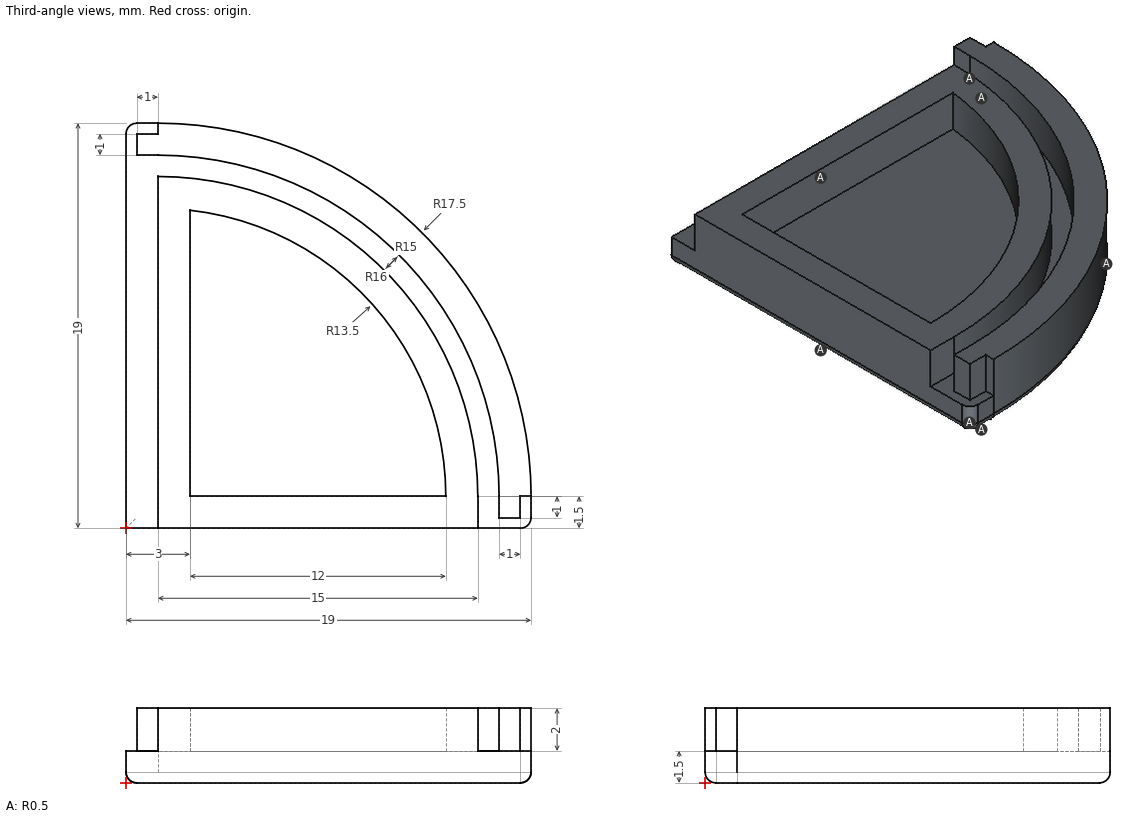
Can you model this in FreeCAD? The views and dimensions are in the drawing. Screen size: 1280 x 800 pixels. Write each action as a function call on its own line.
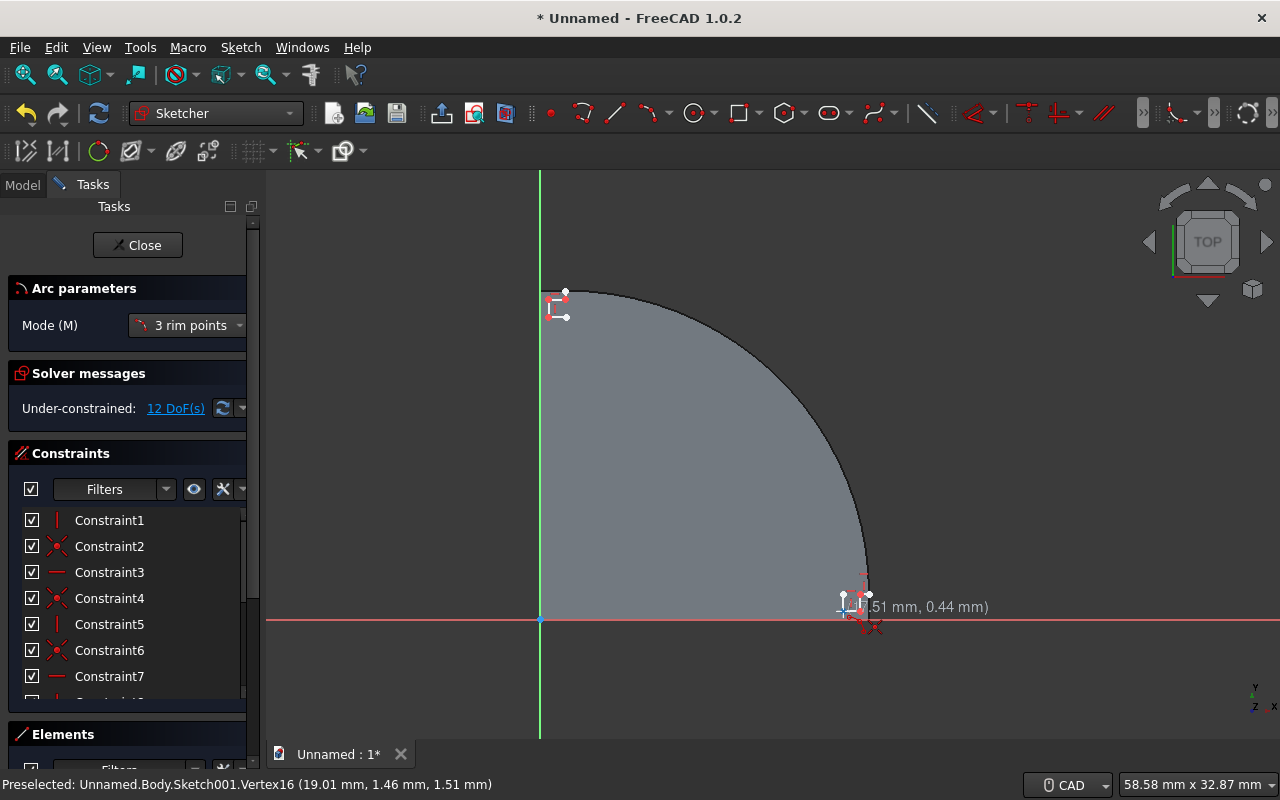
scroll(566, 317, up, 4)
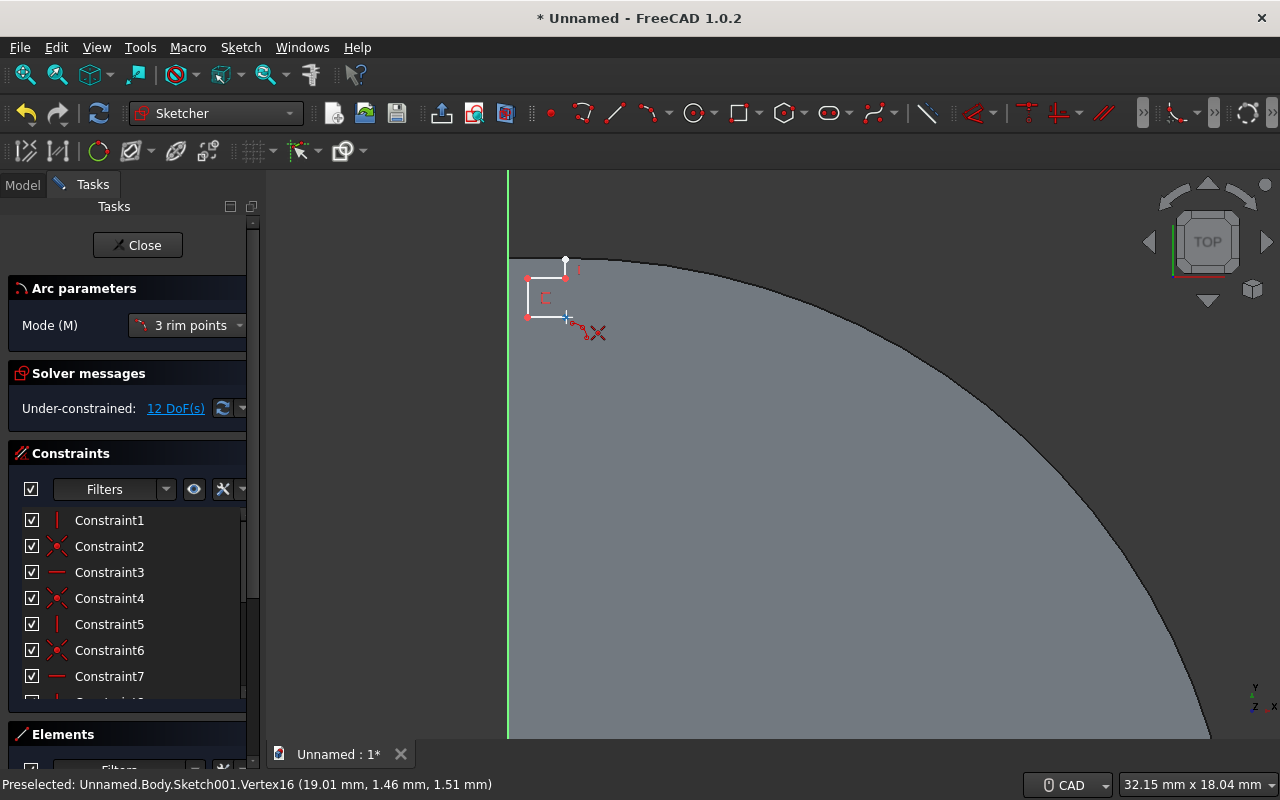
click(566, 317)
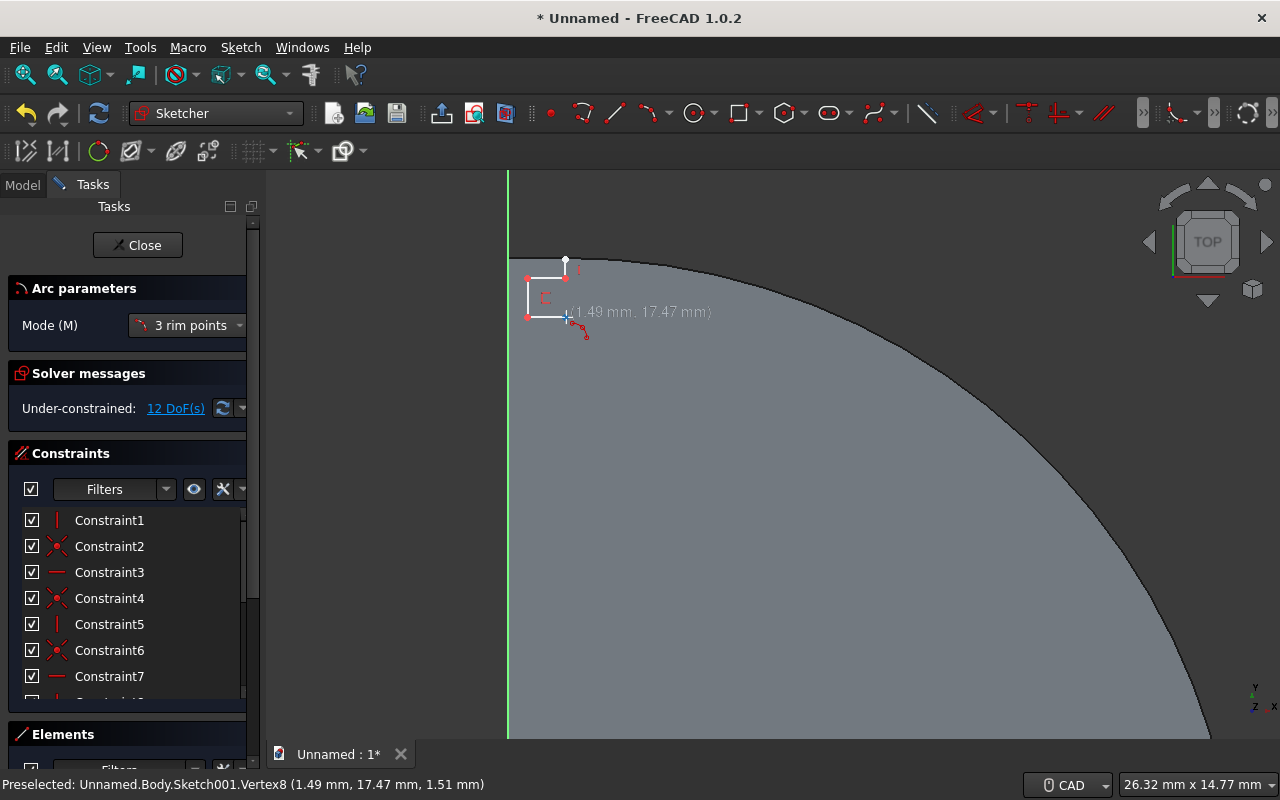
scroll(566, 316, down, 4)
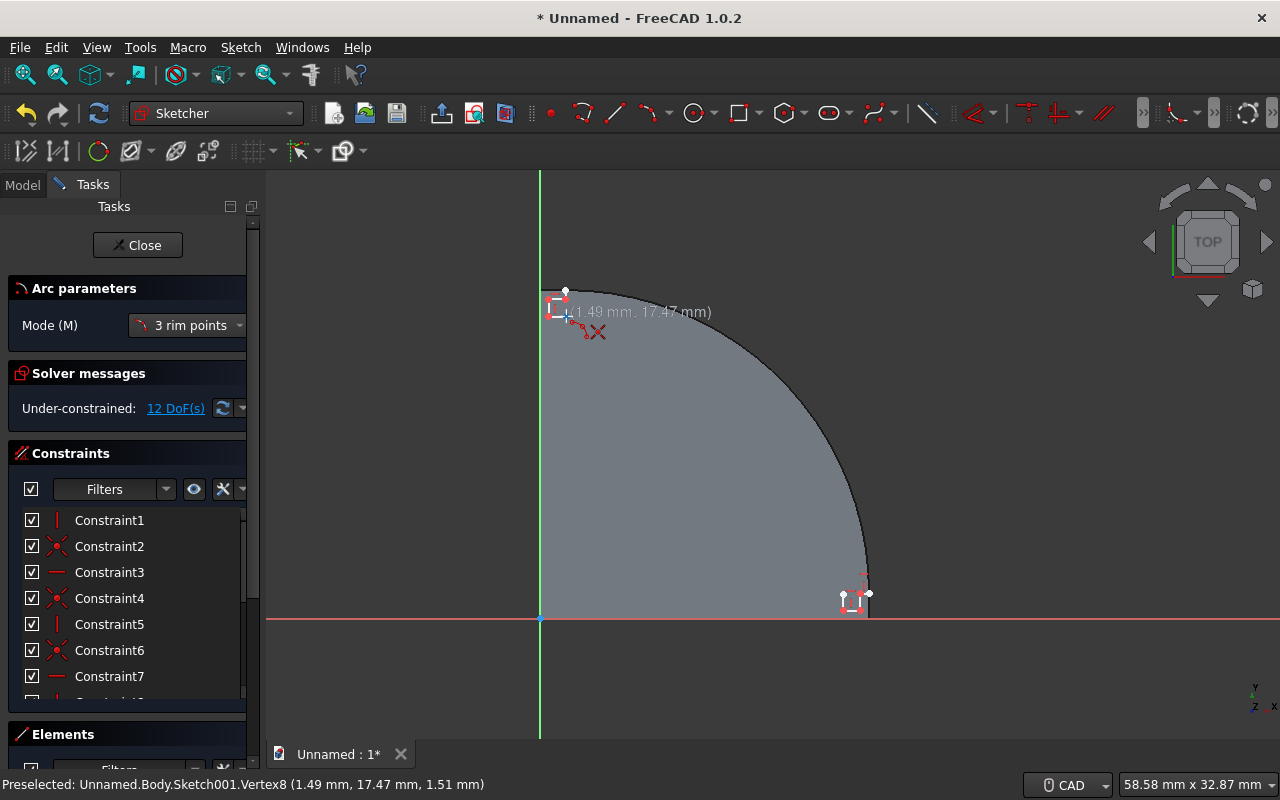
scroll(843, 593, up, 4)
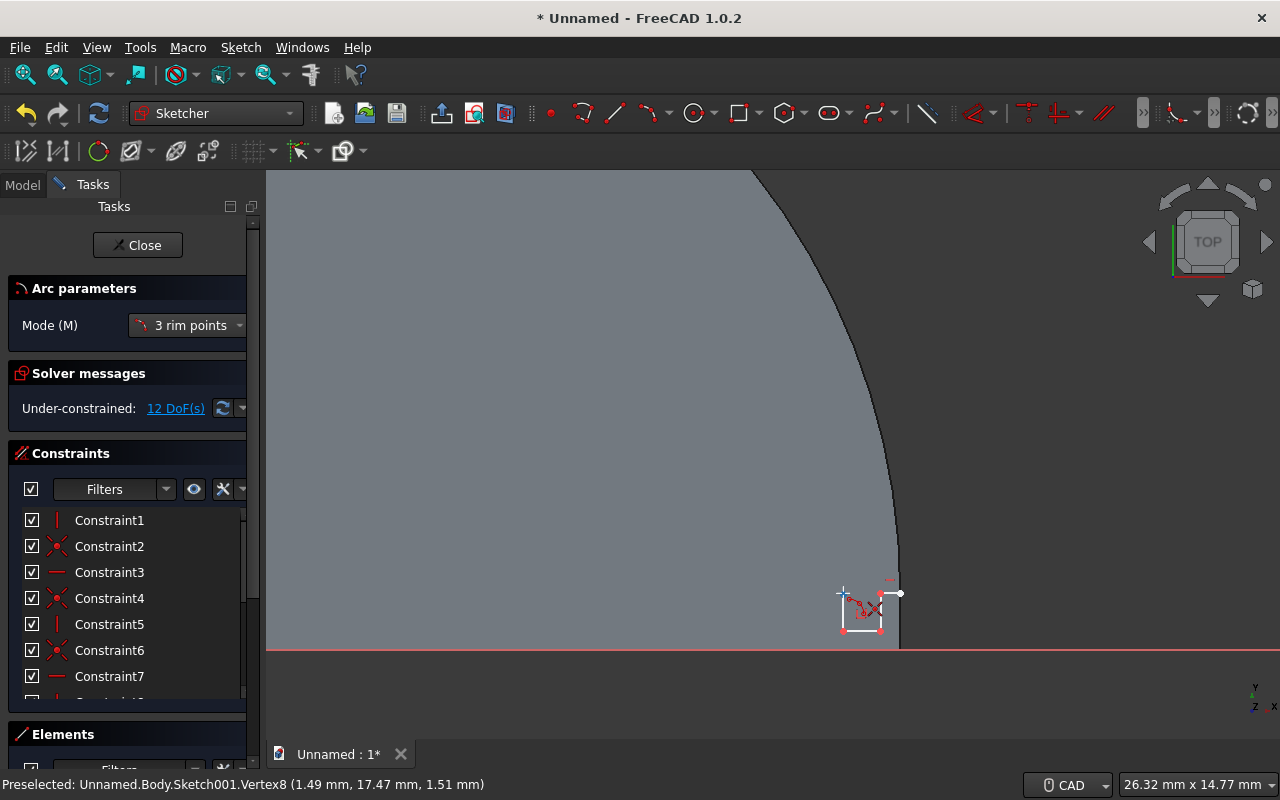
click(843, 595)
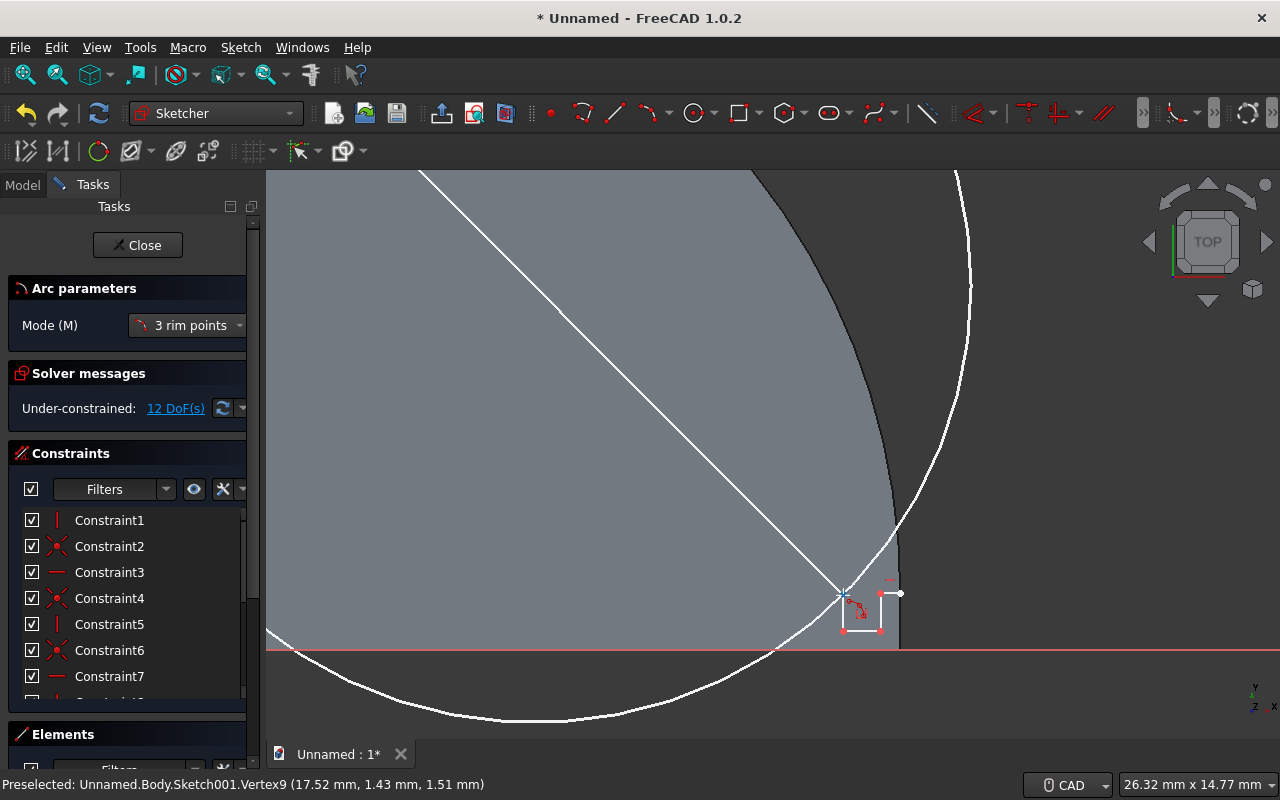
scroll(843, 594, down, 4)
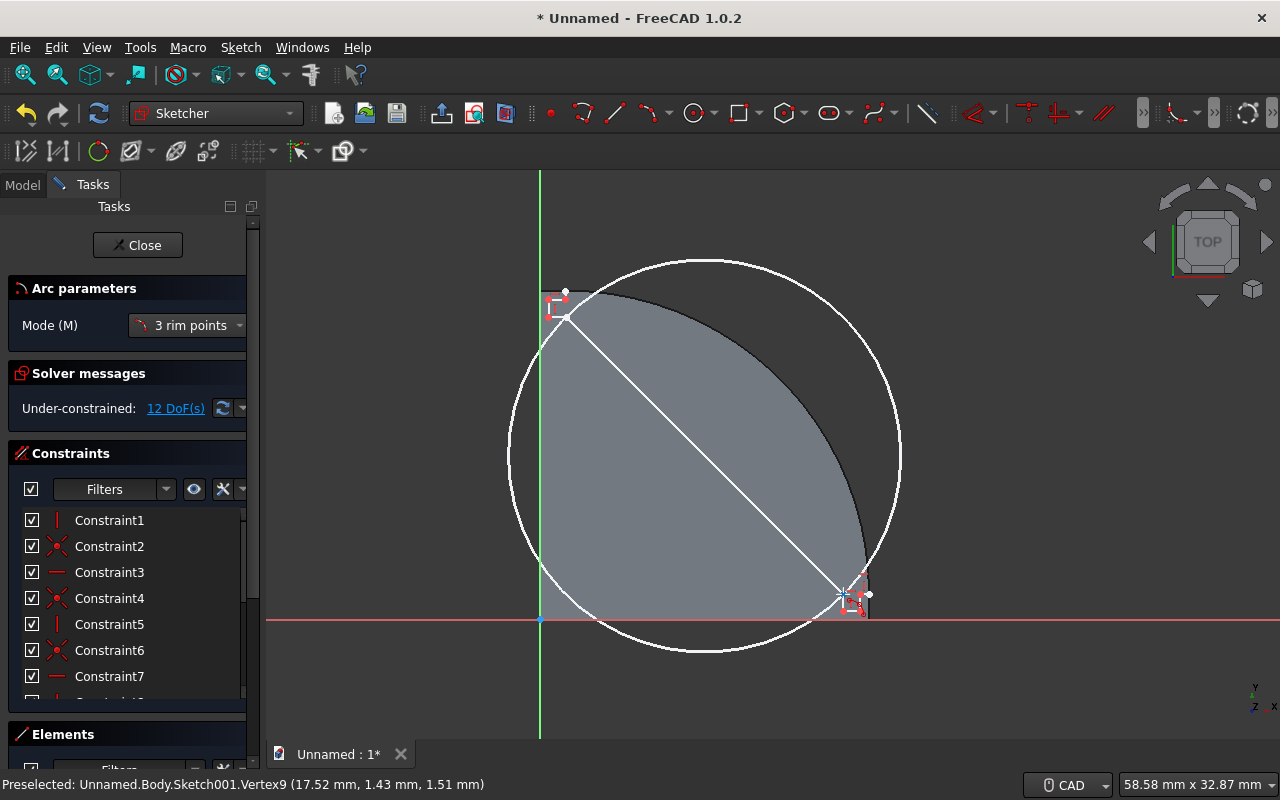
click(762, 398)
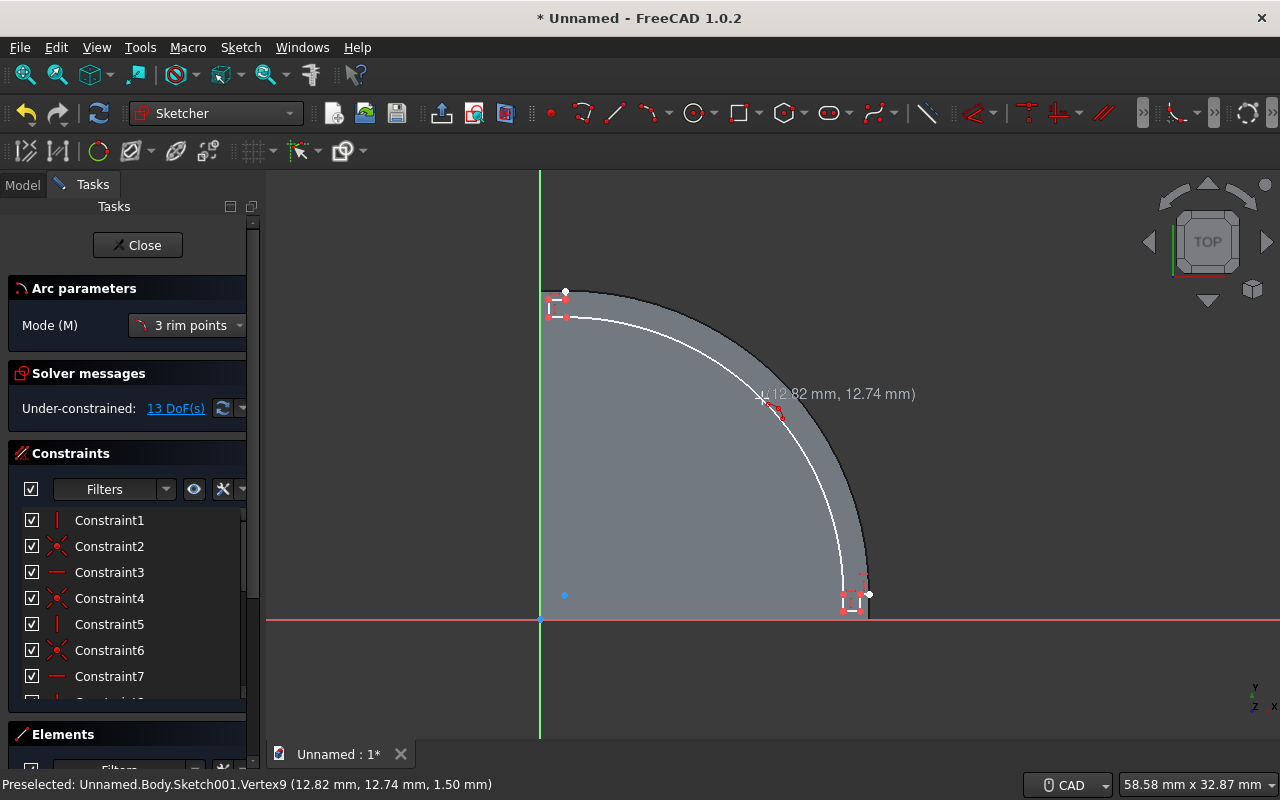
scroll(869, 594, up, 7)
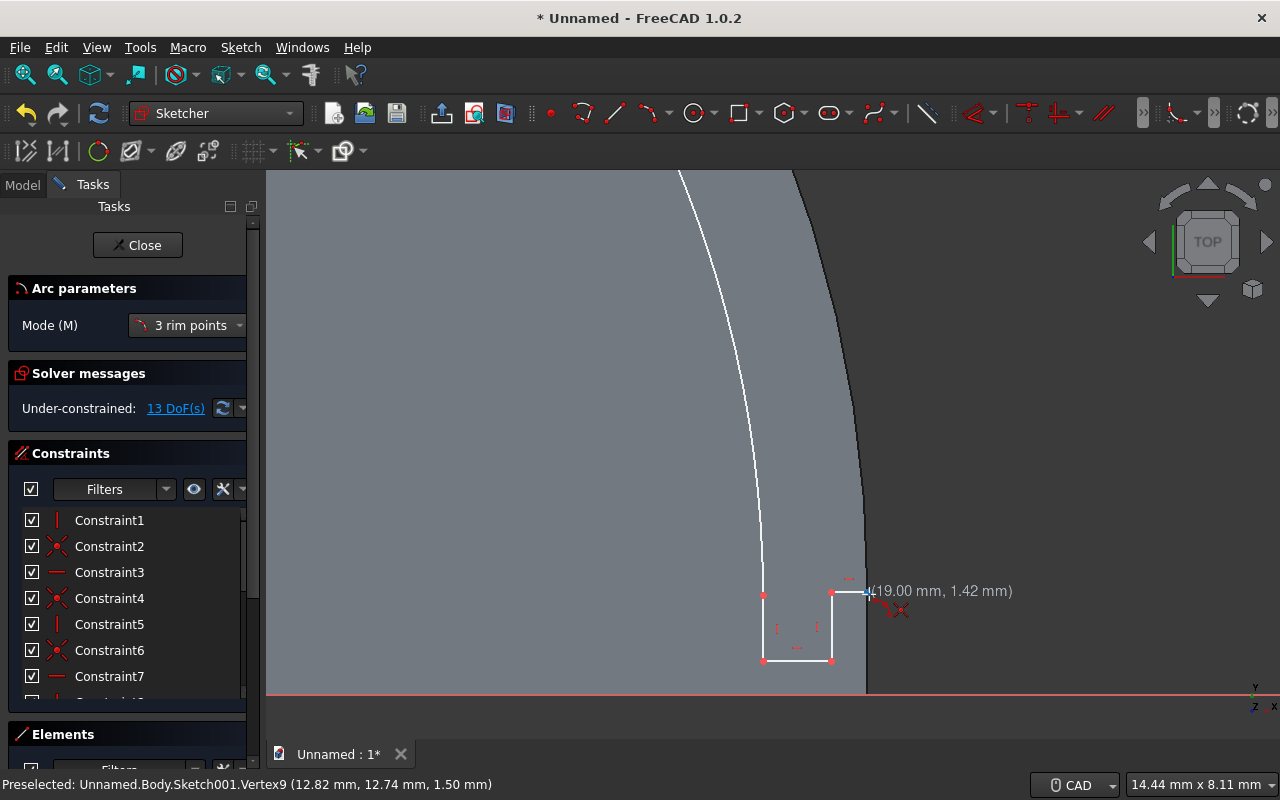
click(868, 592)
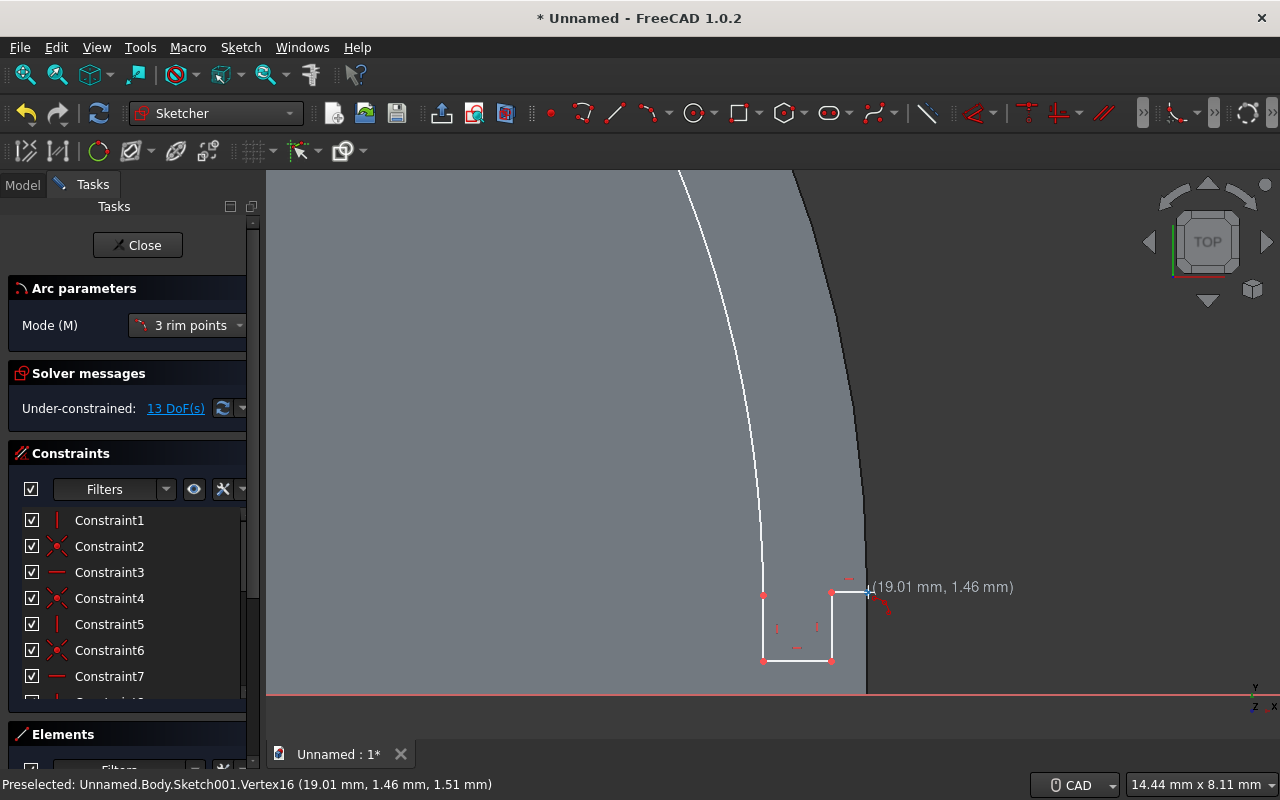
scroll(869, 594, down, 7)